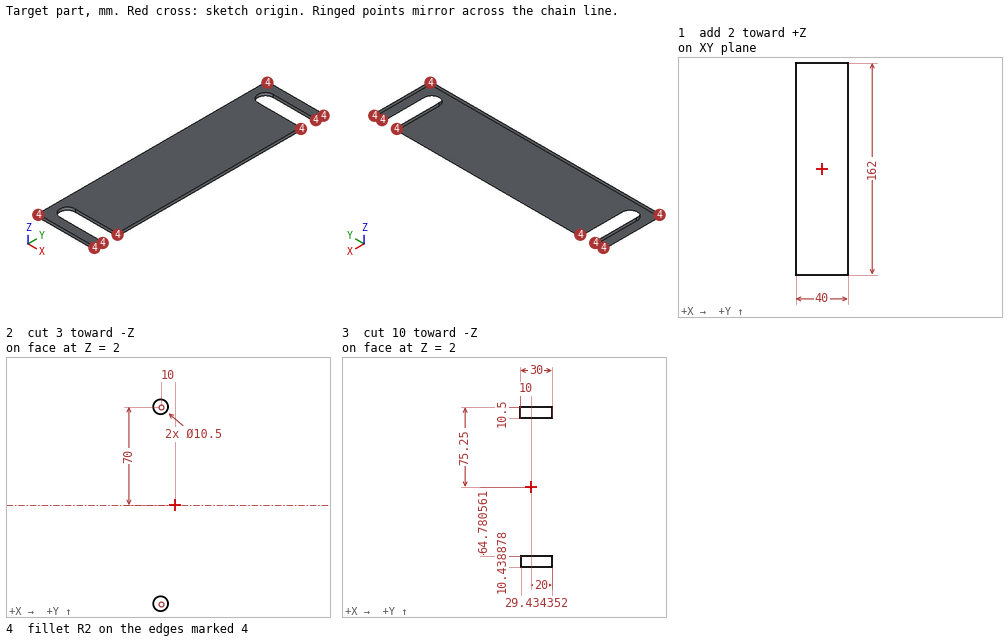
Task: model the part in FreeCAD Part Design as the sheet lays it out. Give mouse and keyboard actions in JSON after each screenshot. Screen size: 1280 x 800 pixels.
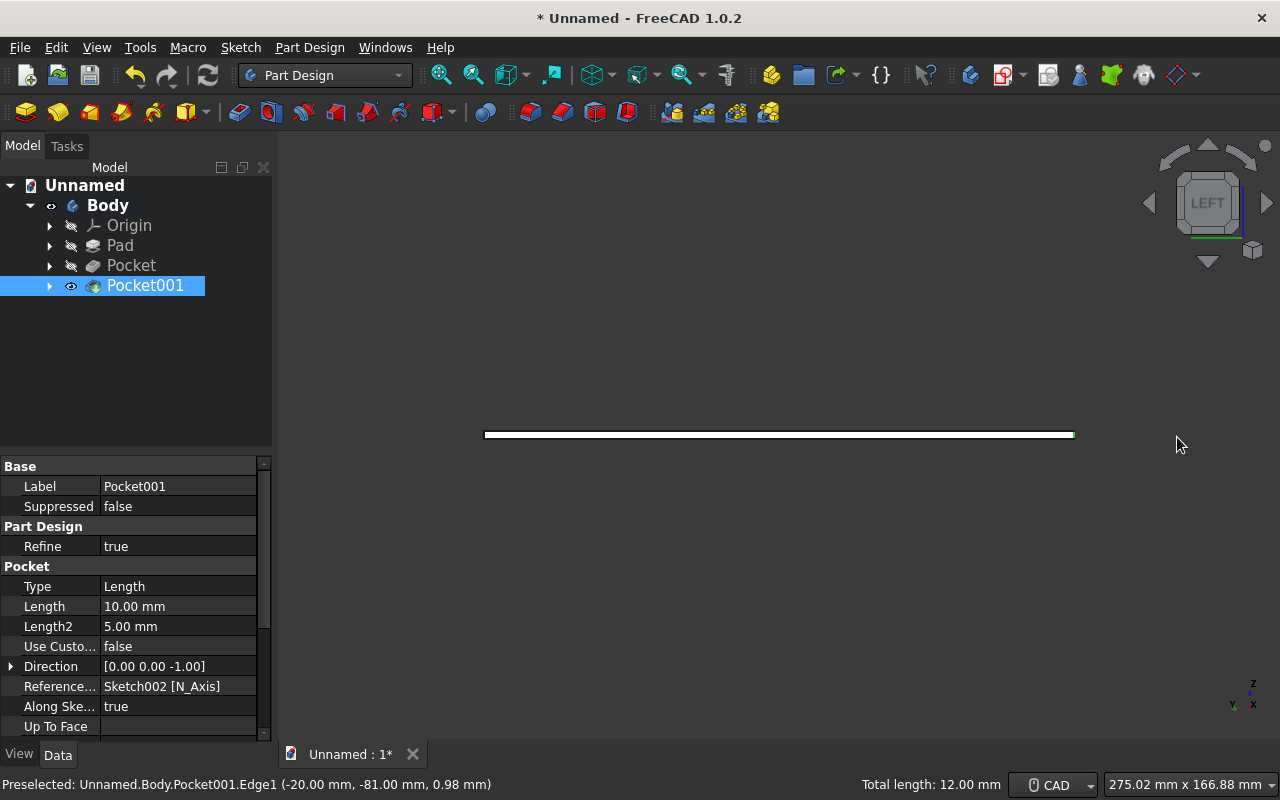
{"action": "key", "text": "0"}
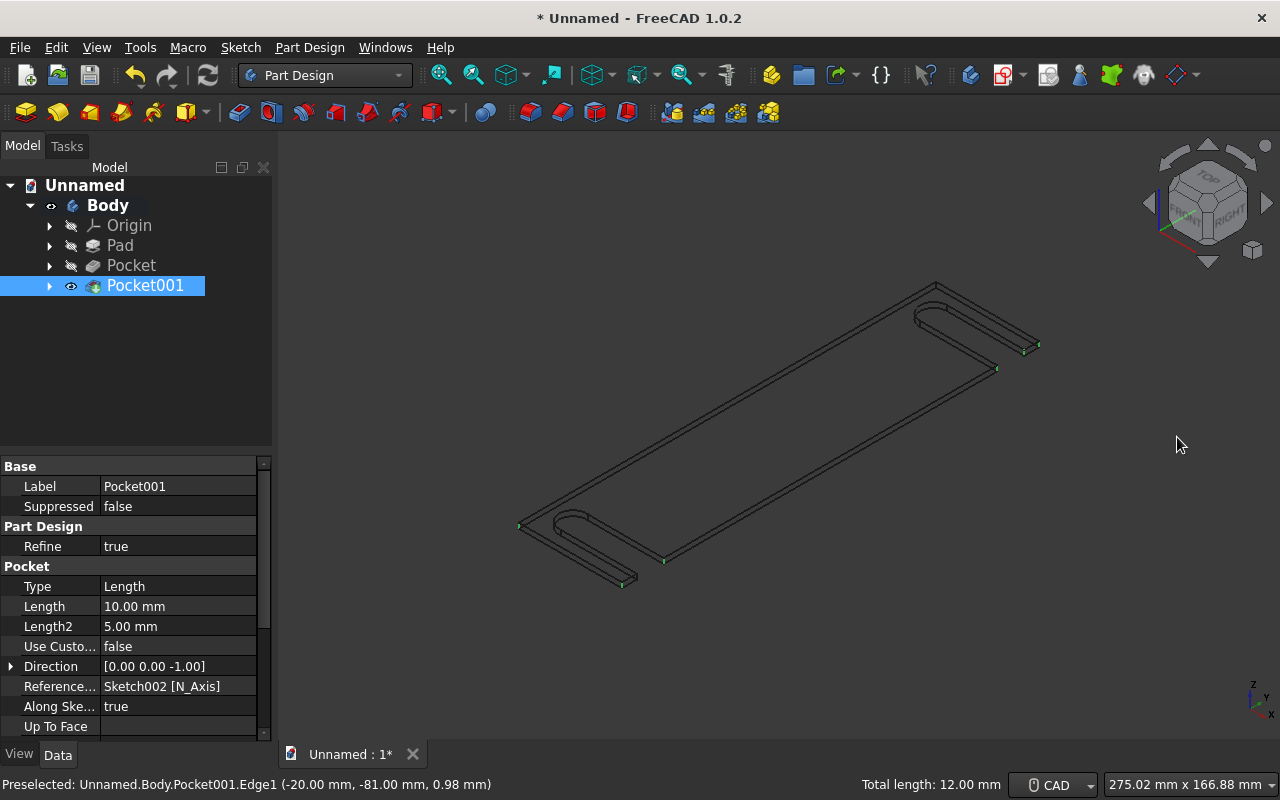
{"action": "scroll", "coordinate": [637, 576], "scroll_direction": "up", "scroll_amount": 9}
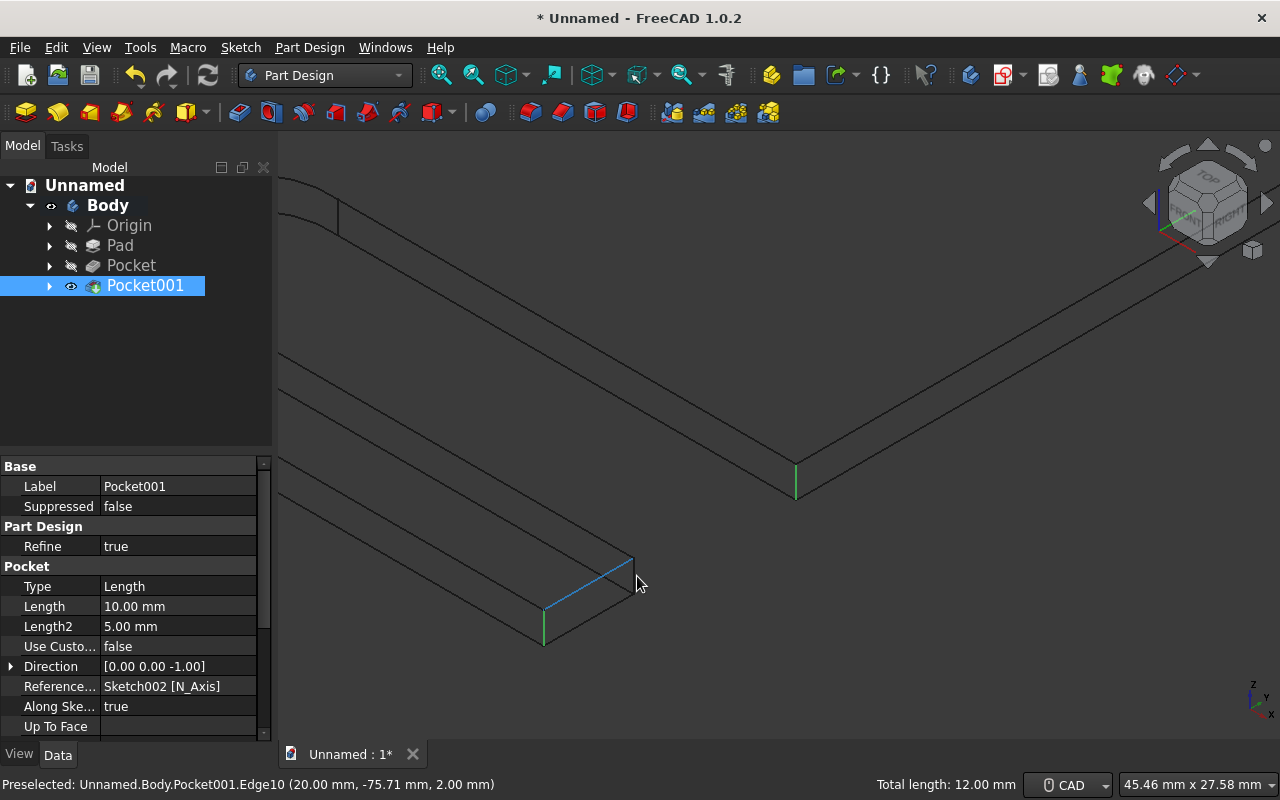
{"action": "left_click", "coordinate": [634, 575], "text": "ctrl"}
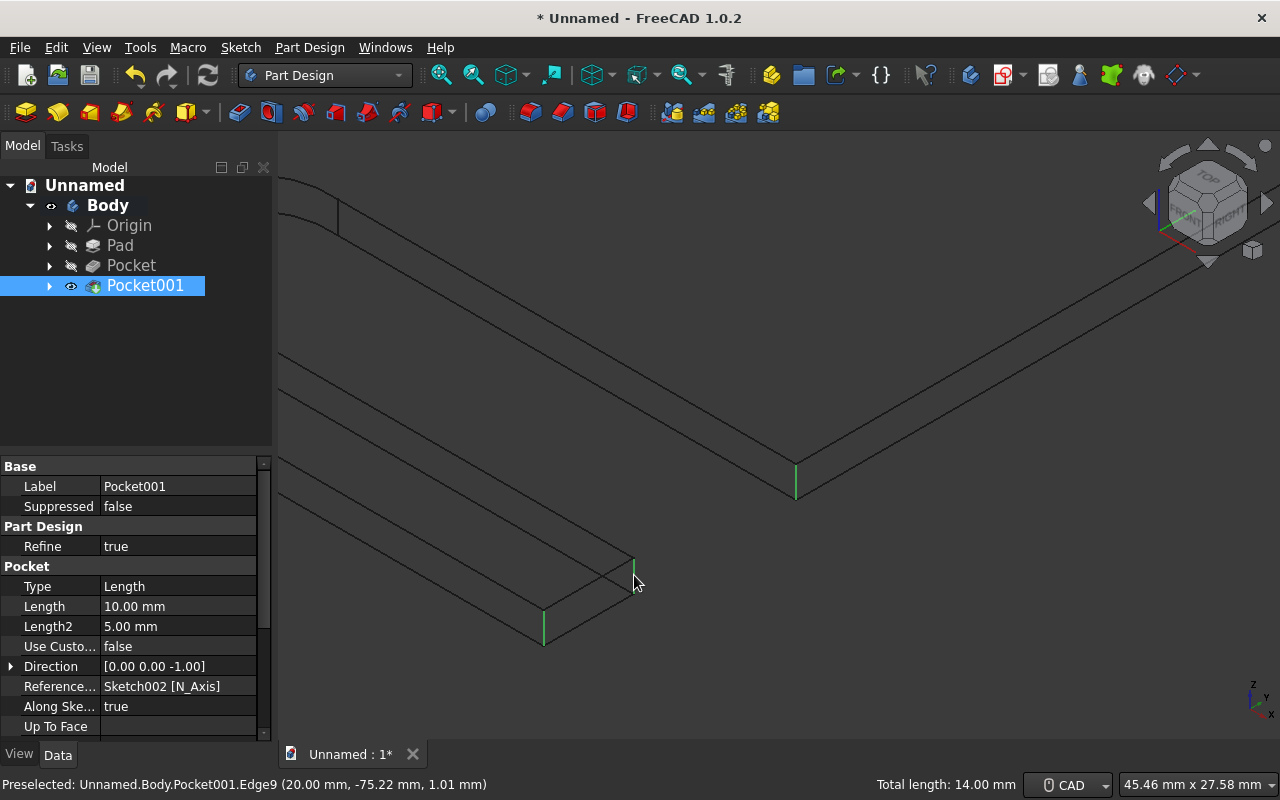
{"action": "left_click", "coordinate": [442, 76]}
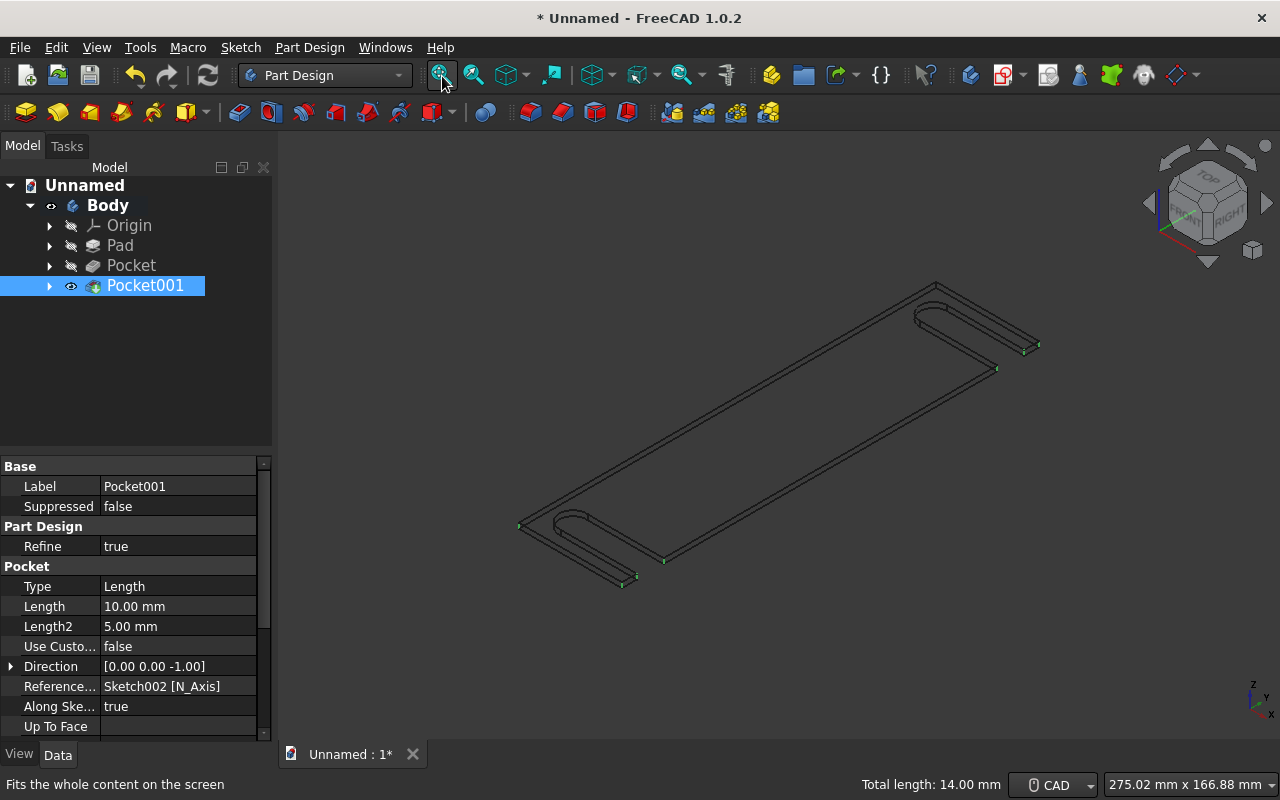
{"action": "key", "text": "2"}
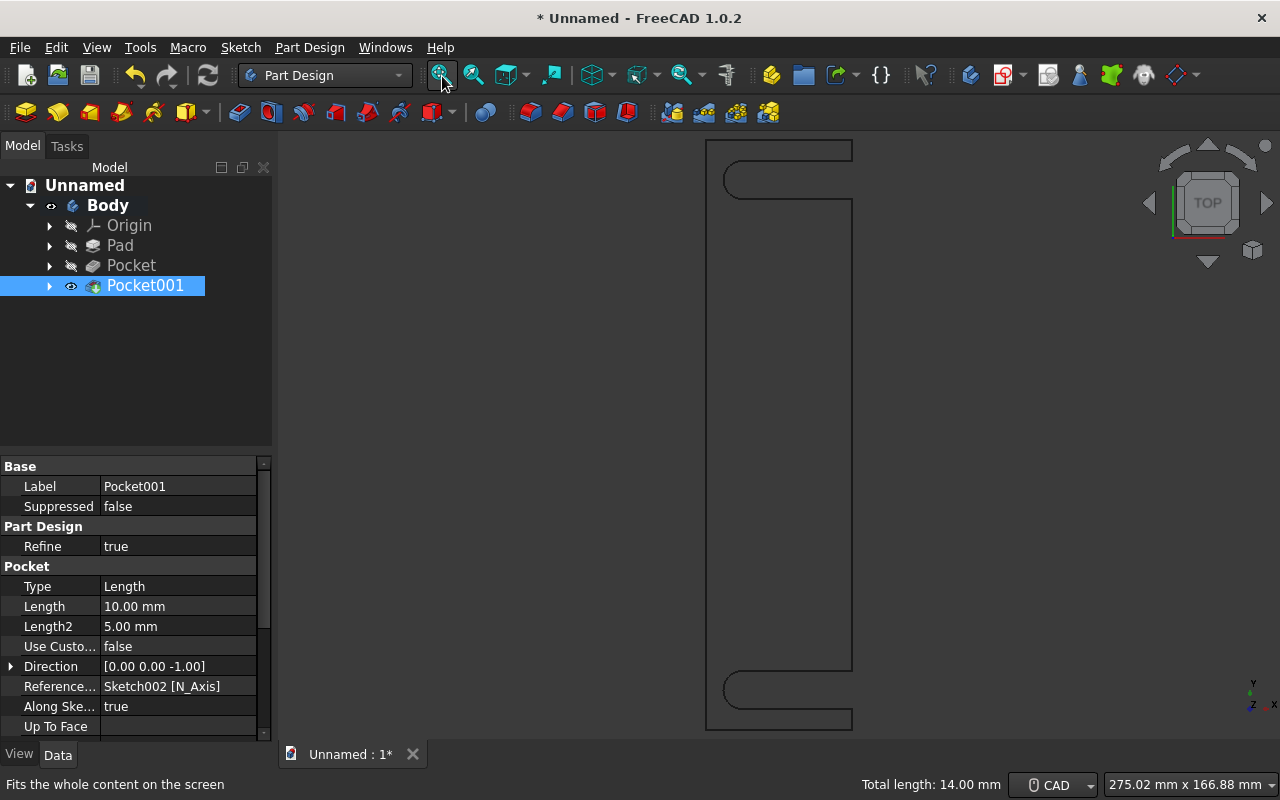
{"action": "key", "text": "1"}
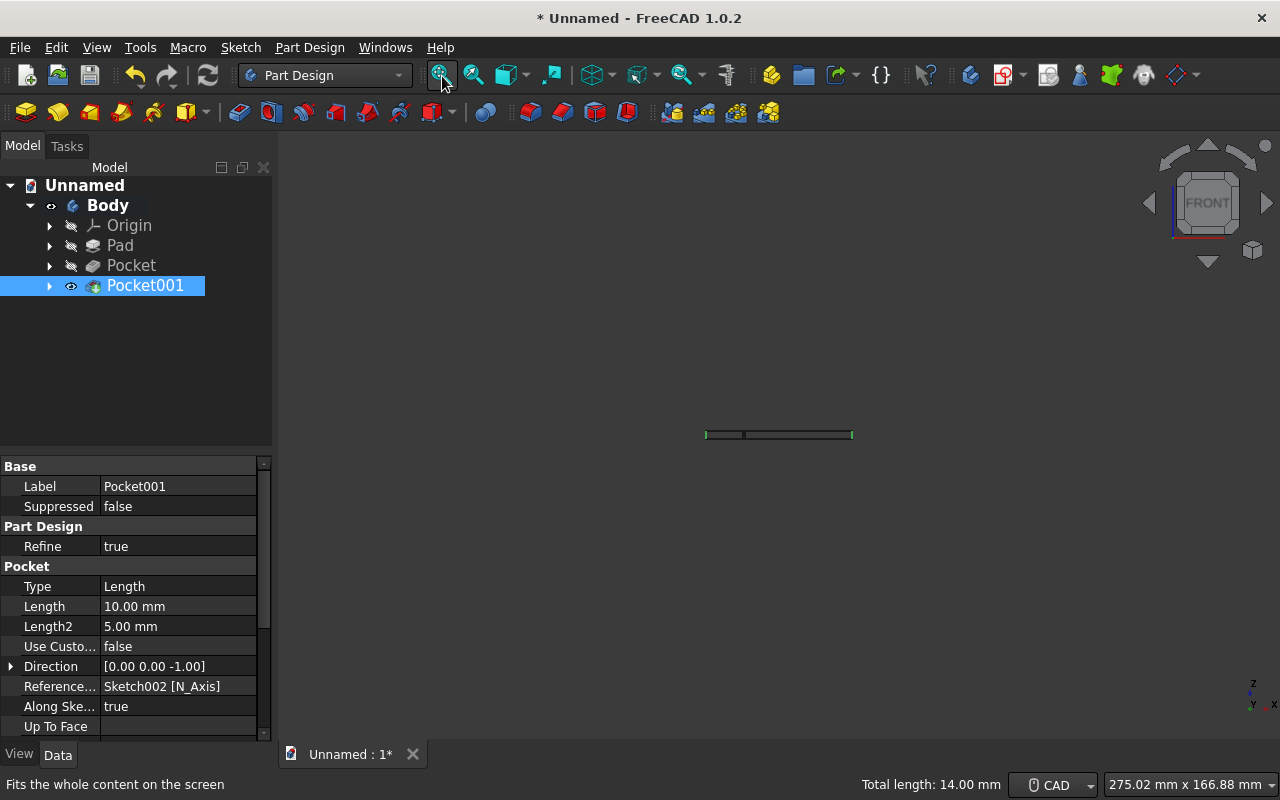
{"action": "key", "text": "v f"}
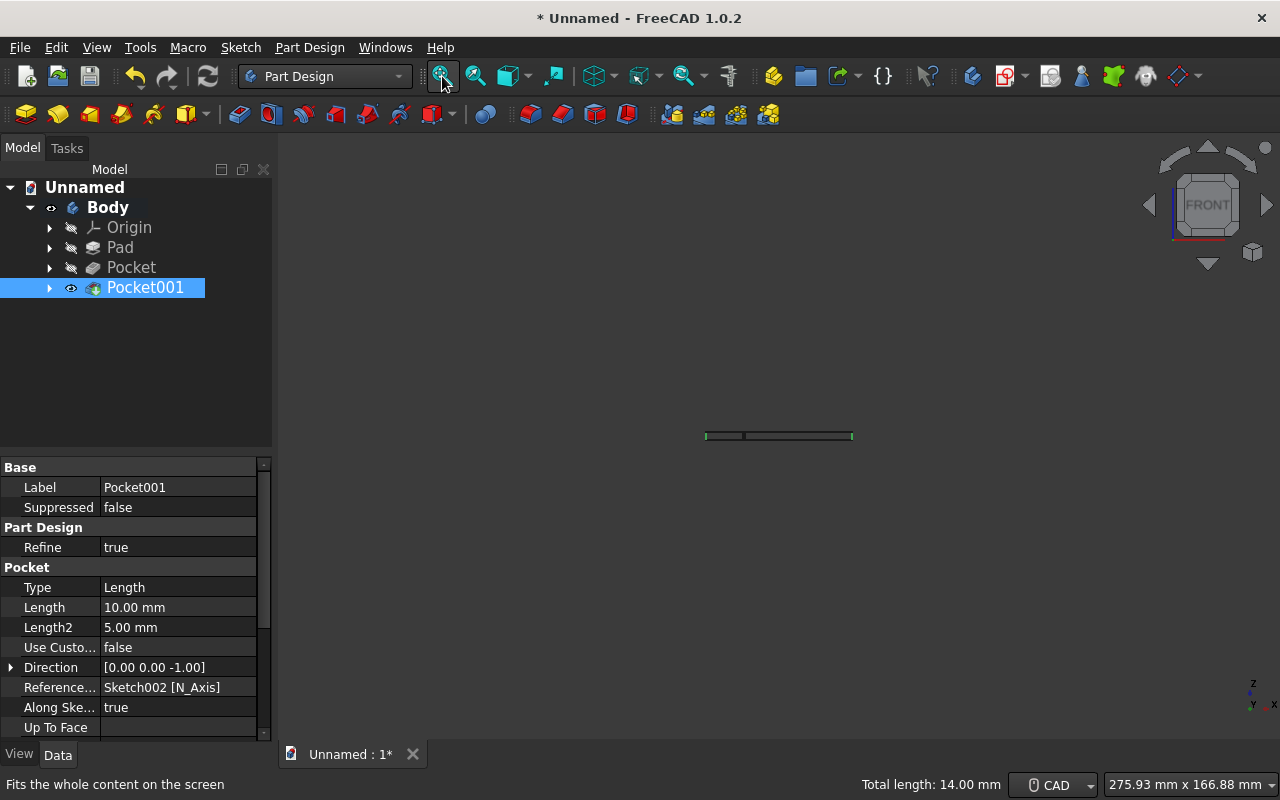
{"action": "scroll", "coordinate": [706, 435], "scroll_direction": "up", "scroll_amount": 9}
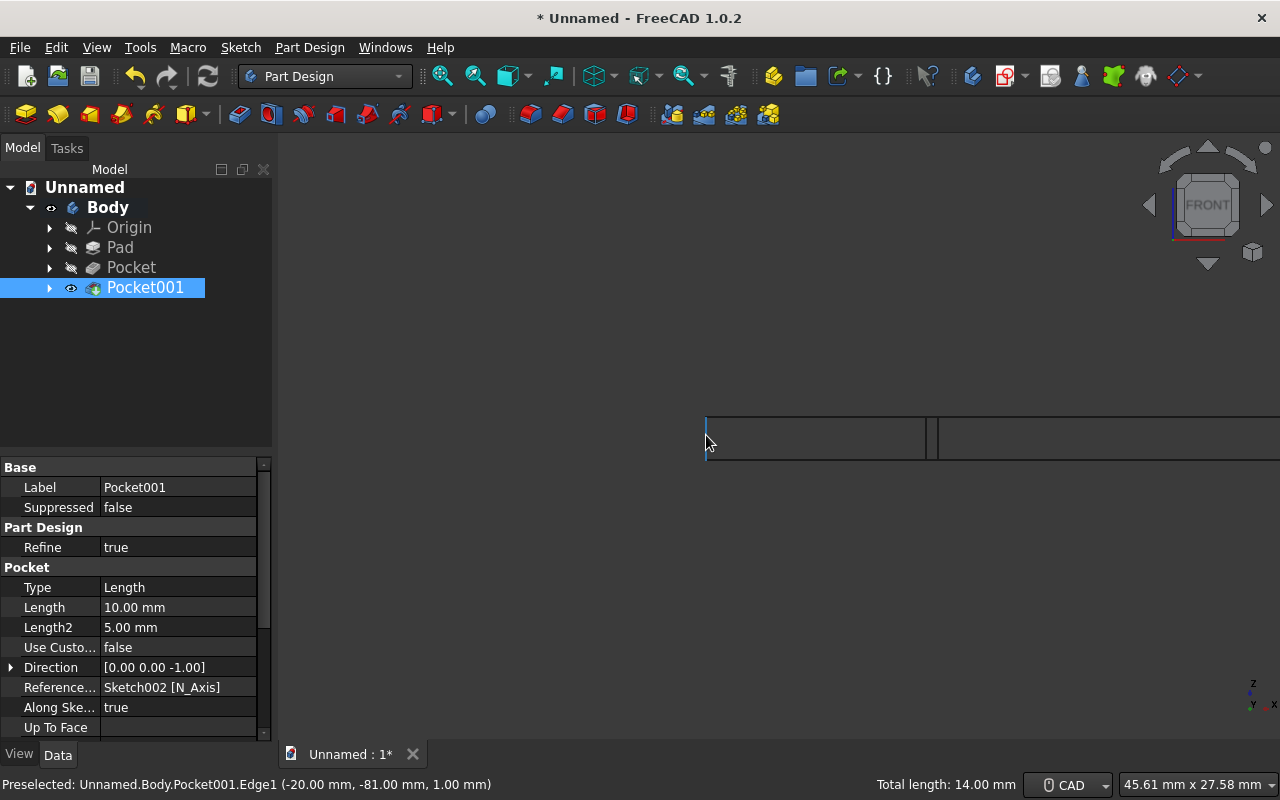
{"action": "left_click", "coordinate": [444, 76]}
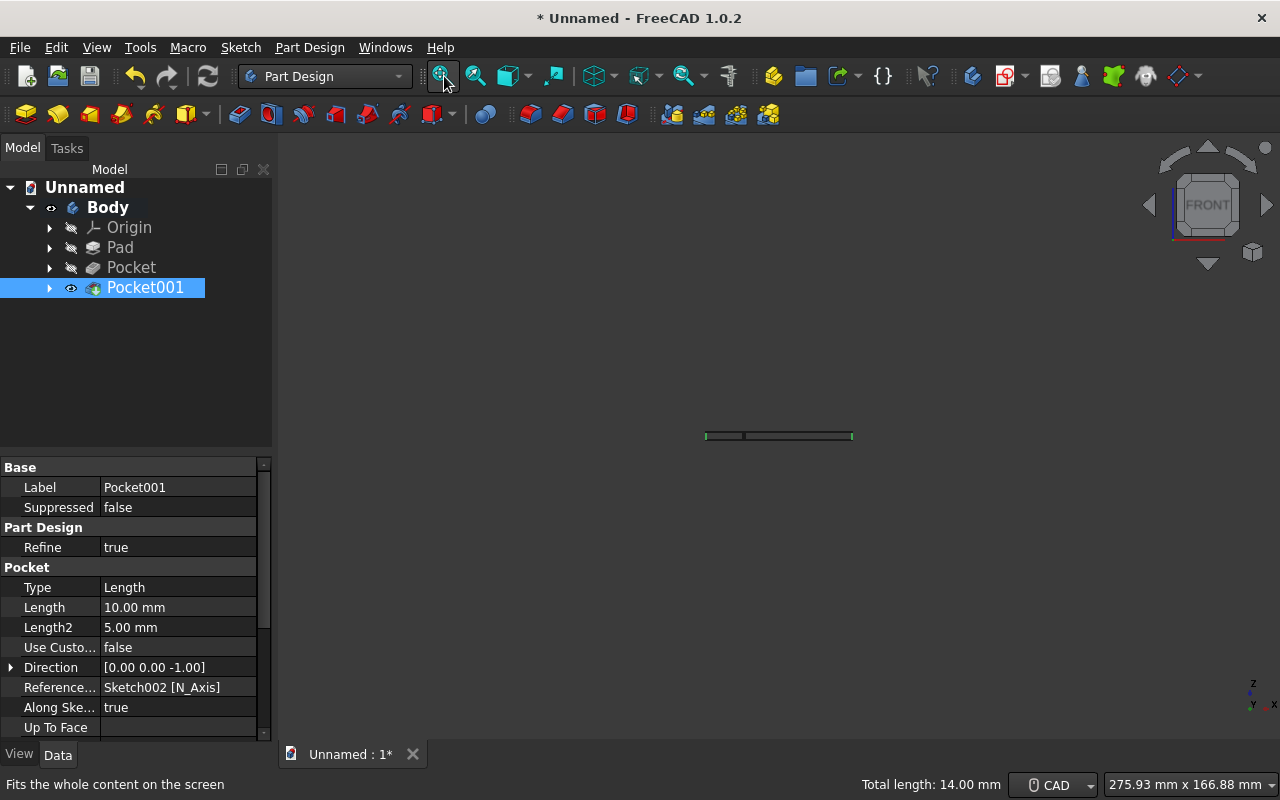
{"action": "key", "text": "3"}